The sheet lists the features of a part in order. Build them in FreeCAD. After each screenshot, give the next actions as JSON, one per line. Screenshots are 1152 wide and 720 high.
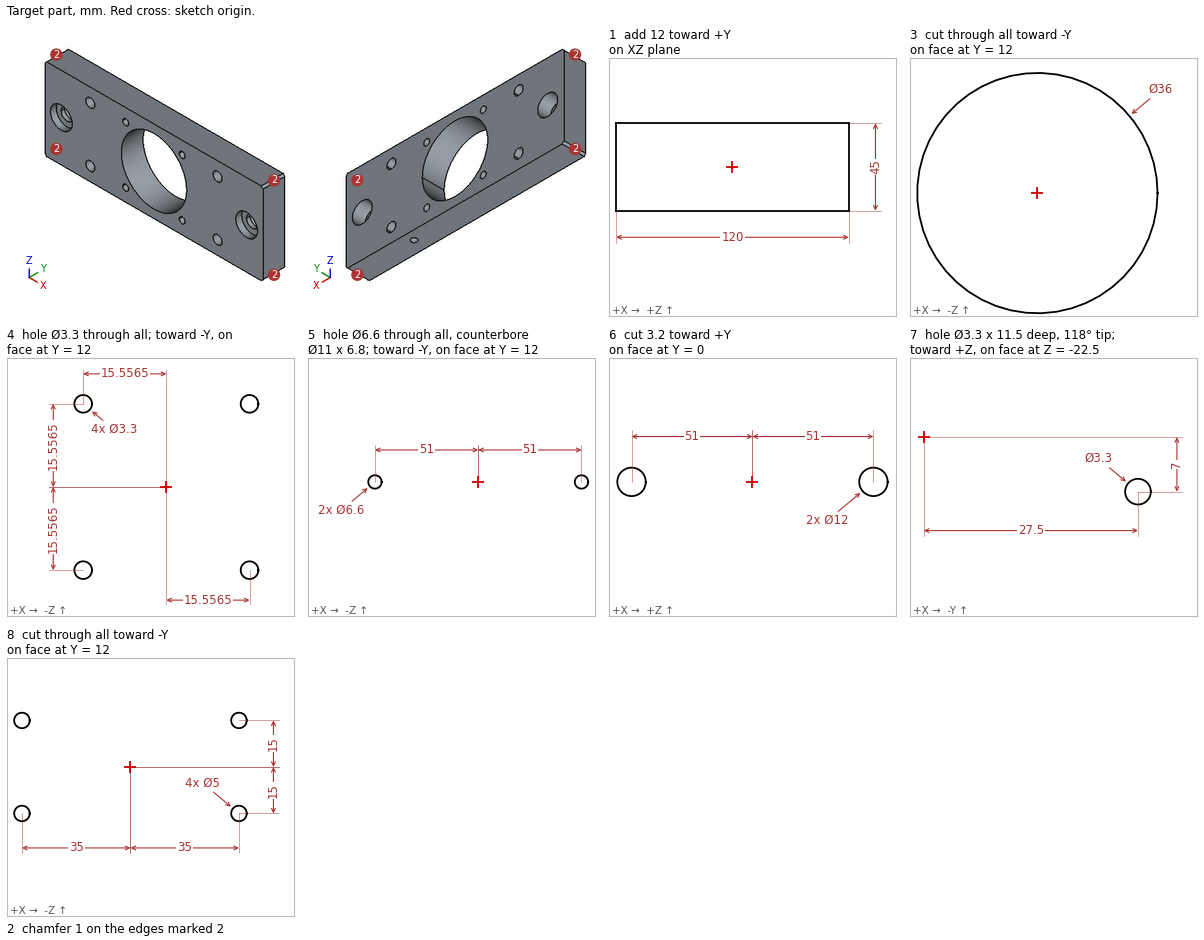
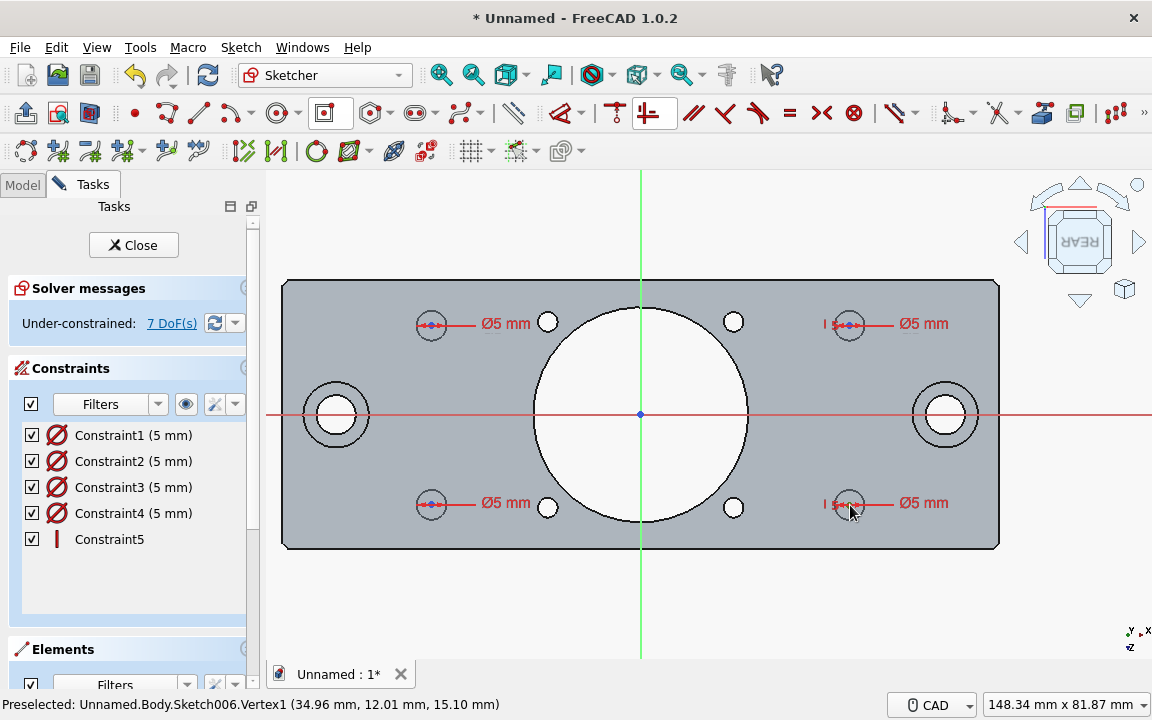
{"action": "left_click", "coordinate": [432, 505]}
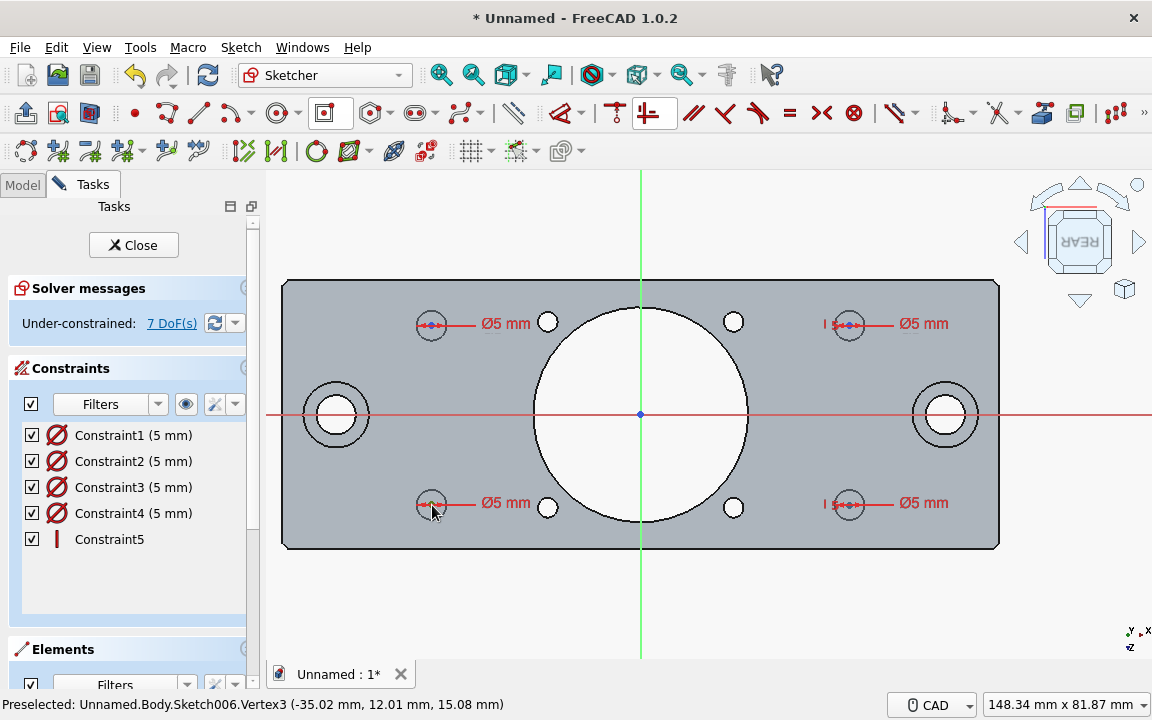
{"action": "key", "text": "h"}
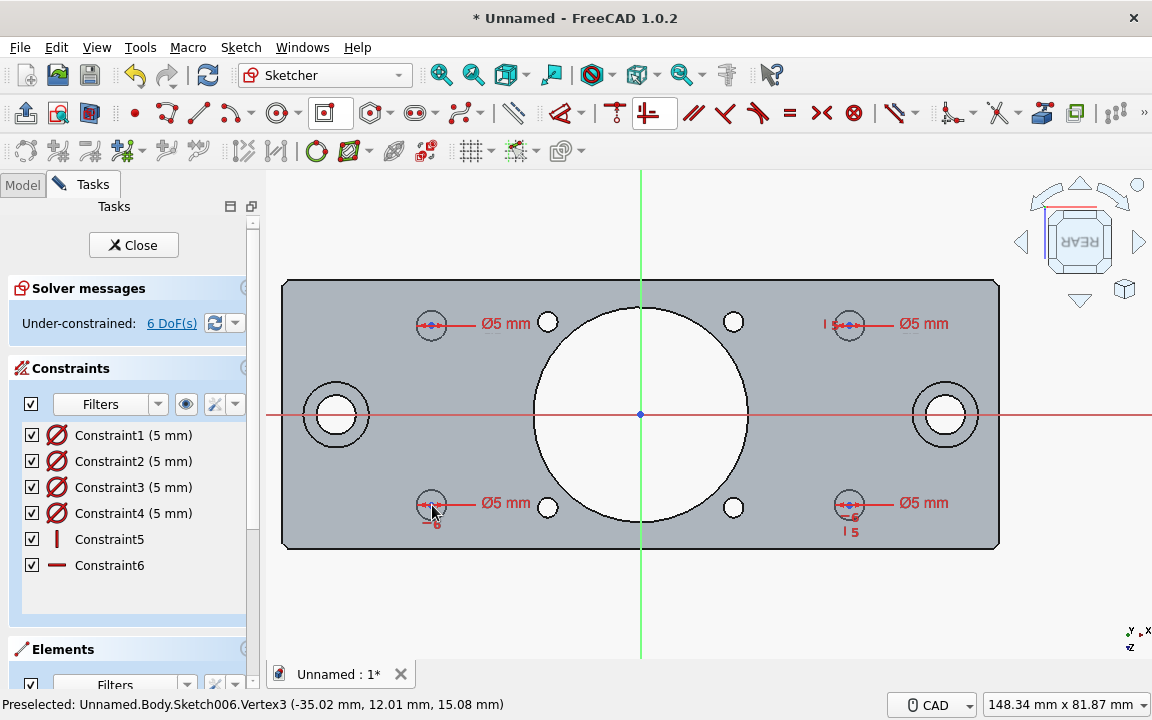
{"action": "left_click", "coordinate": [432, 505]}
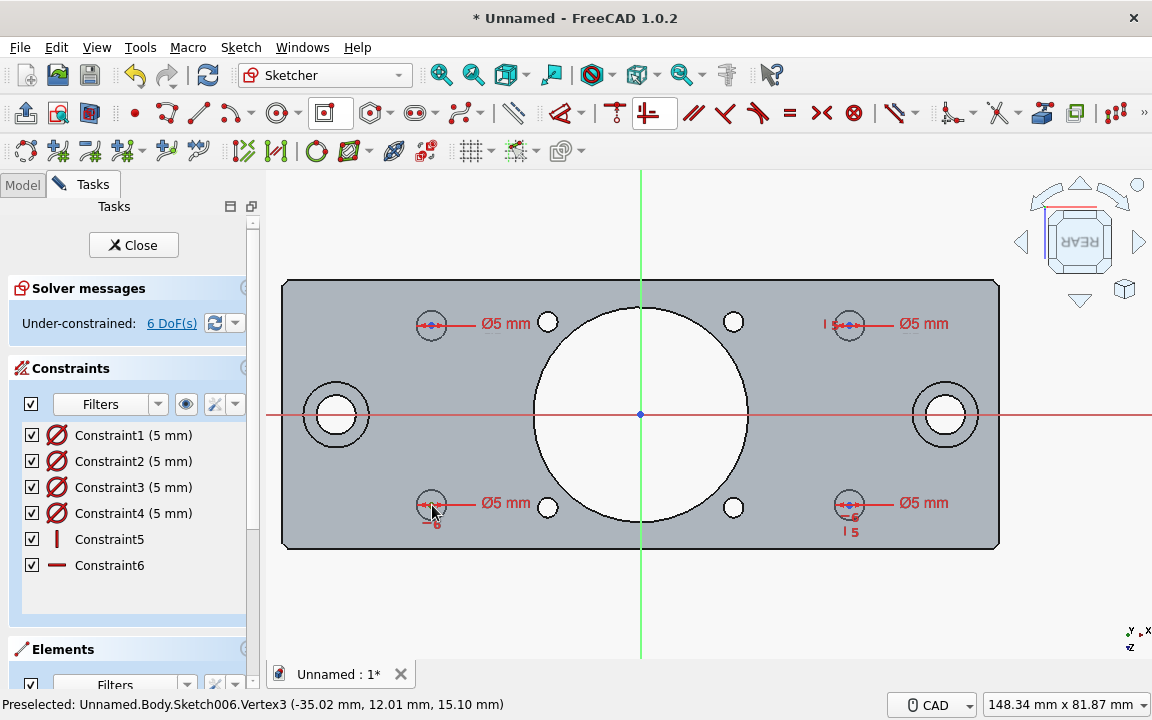
{"action": "left_click", "coordinate": [432, 326]}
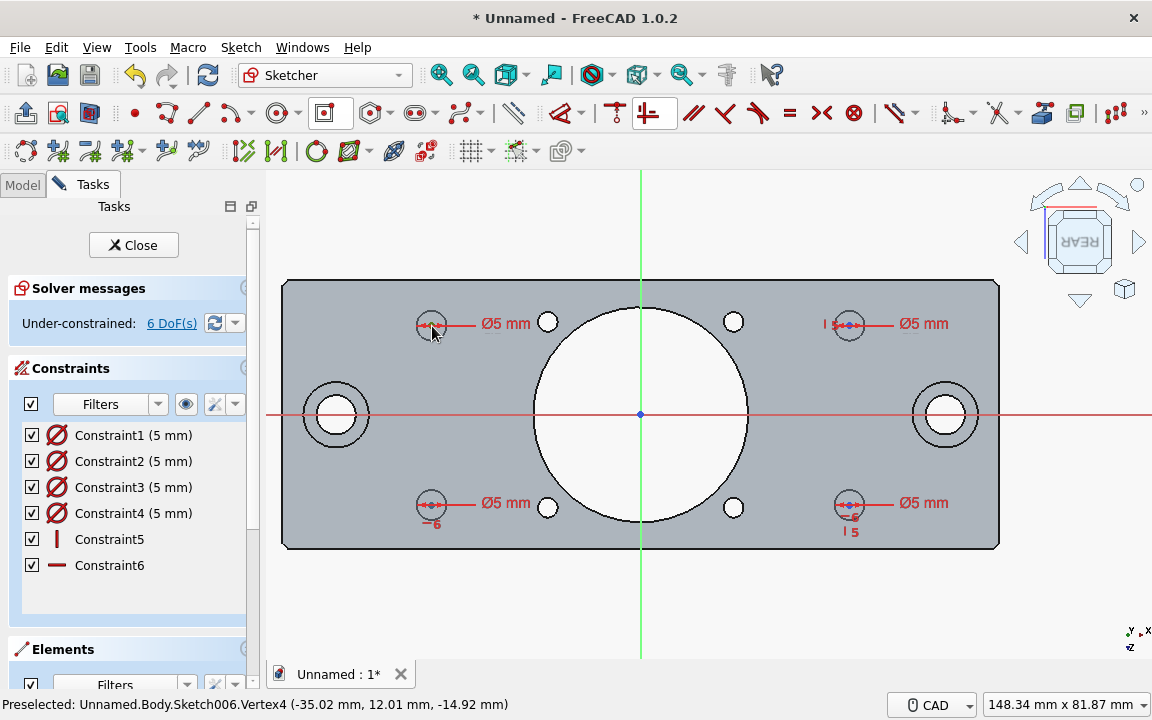
{"action": "key", "text": "v"}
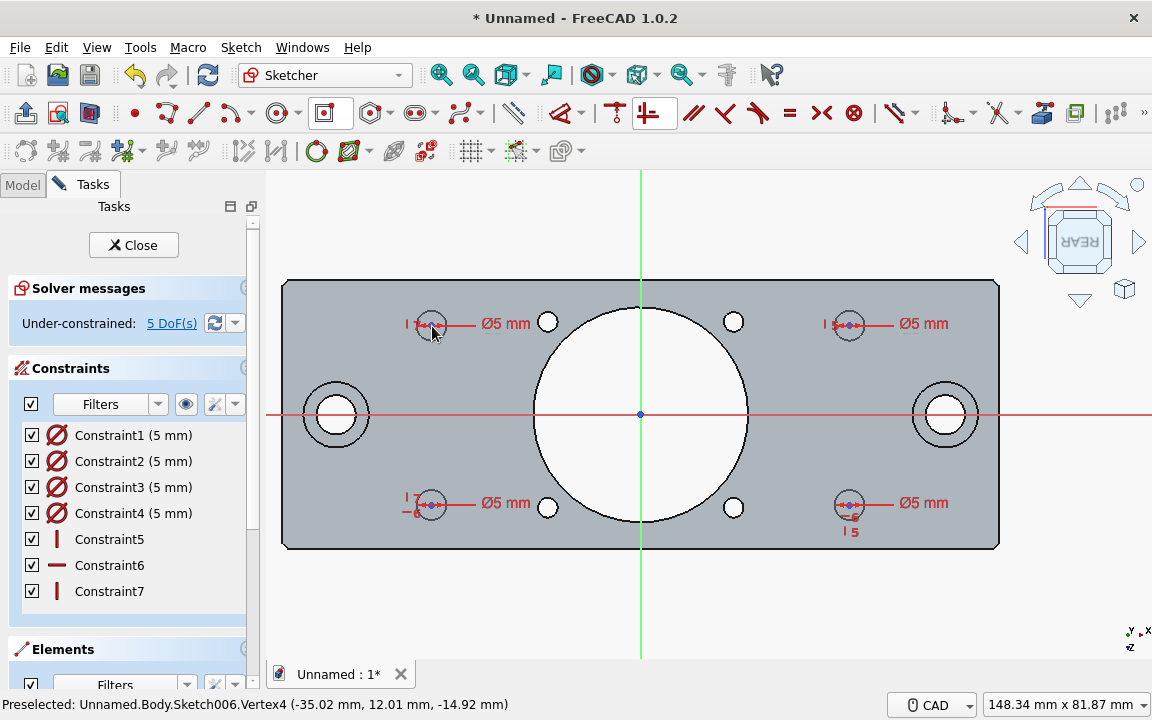
{"action": "left_click", "coordinate": [850, 326]}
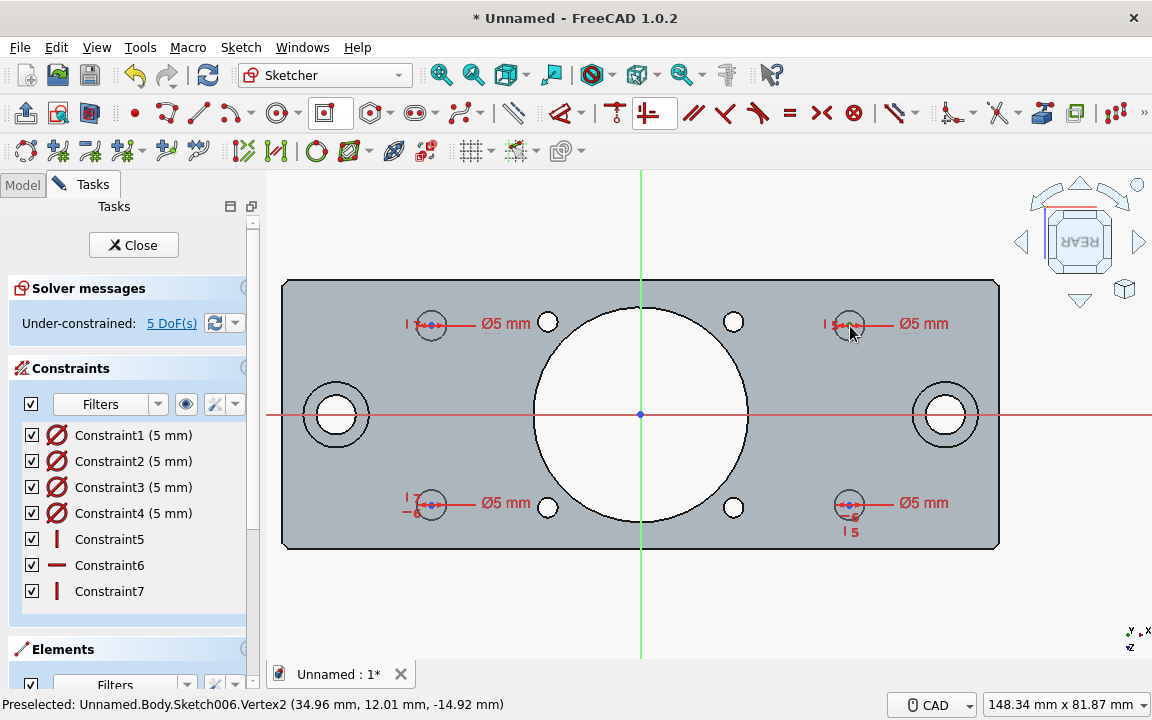
{"action": "left_click", "coordinate": [432, 326]}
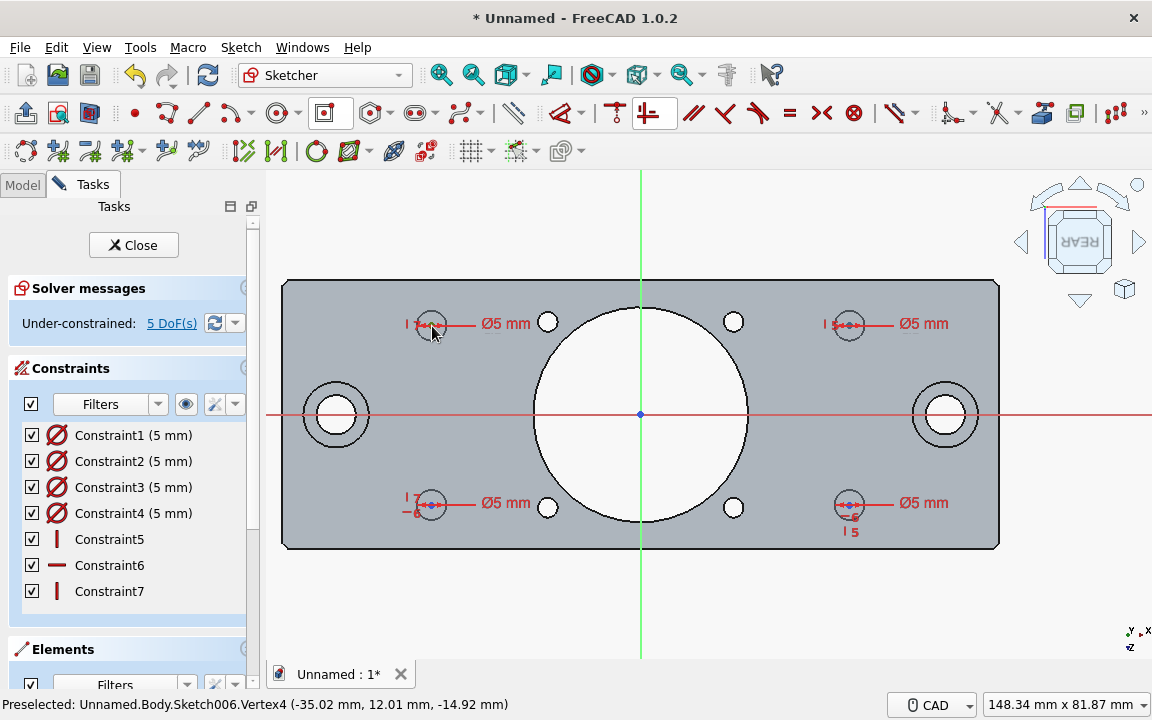
{"action": "left_click", "coordinate": [672, 114]}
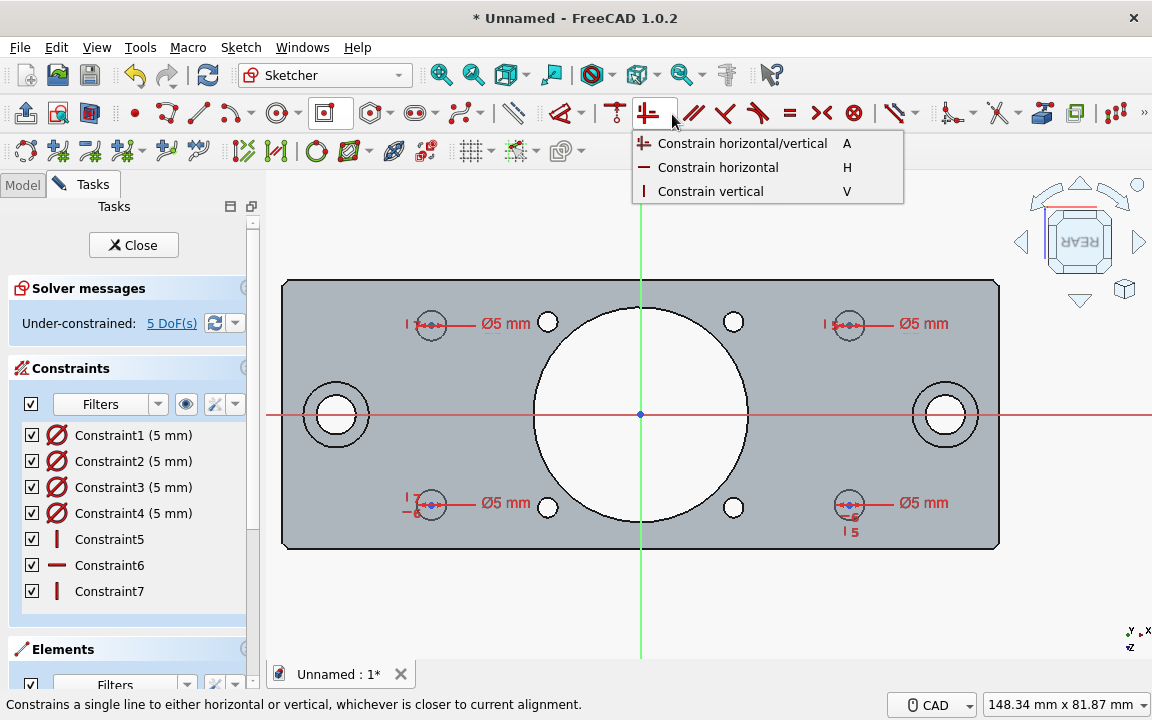
{"action": "left_click", "coordinate": [768, 167]}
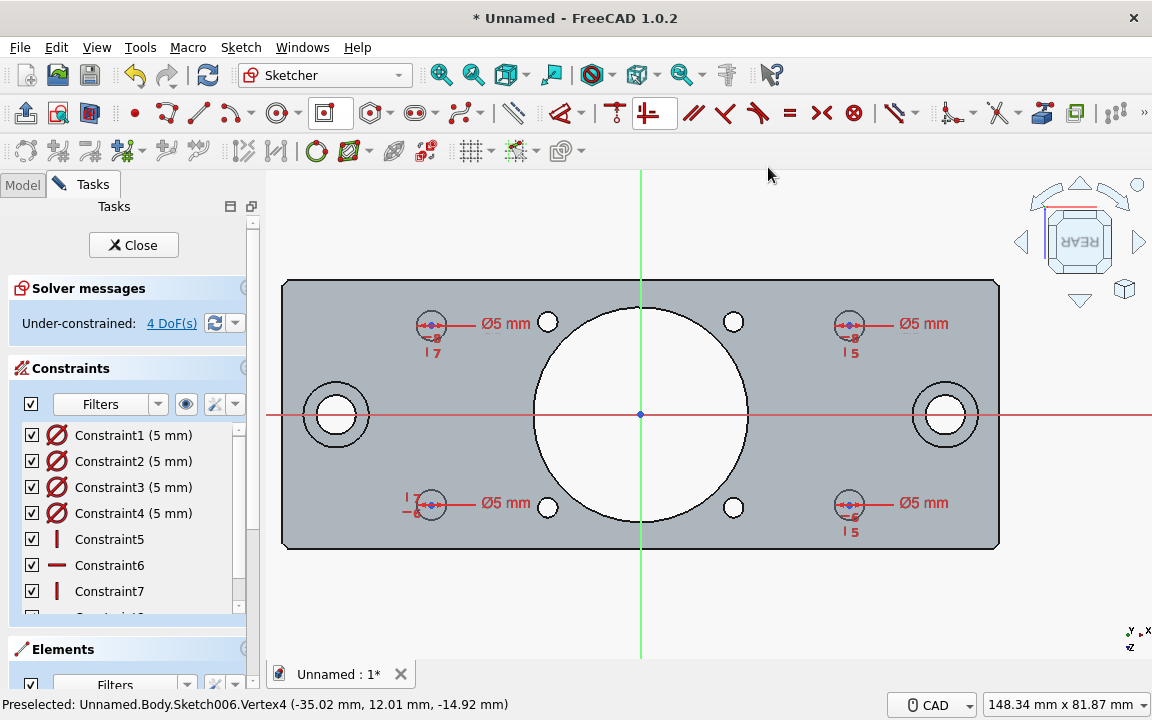
{"action": "left_click", "coordinate": [560, 114]}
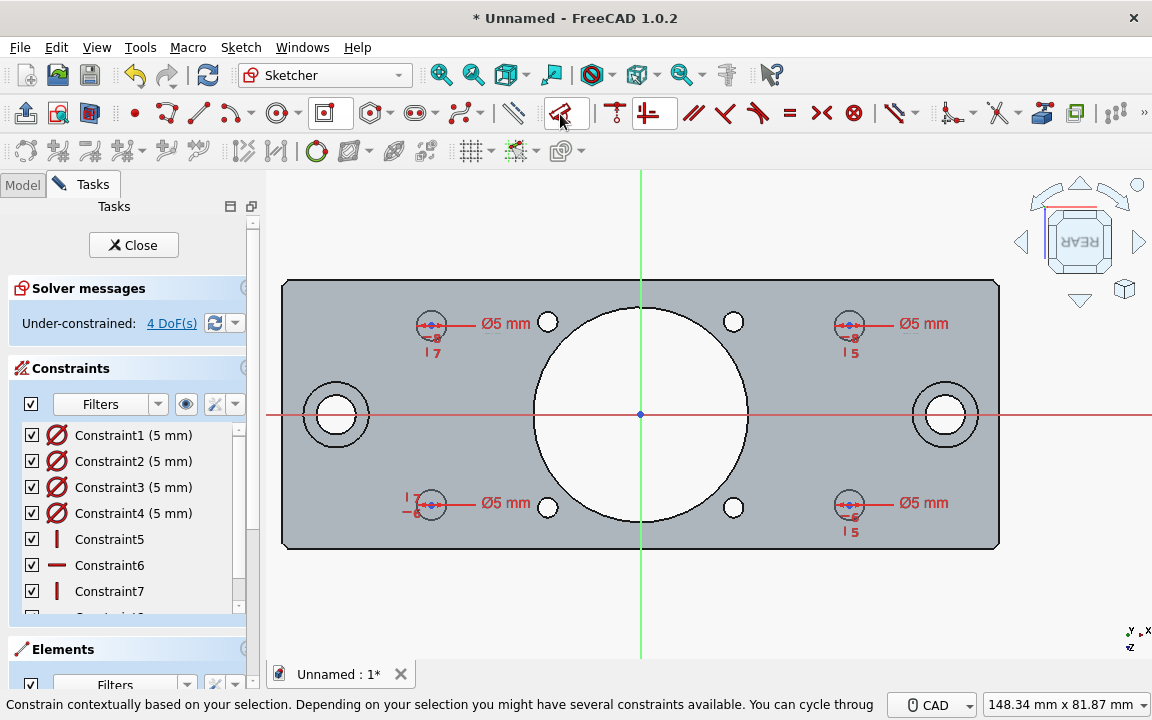
{"action": "left_click", "coordinate": [850, 505]}
{"action": "left_click", "coordinate": [745, 539]}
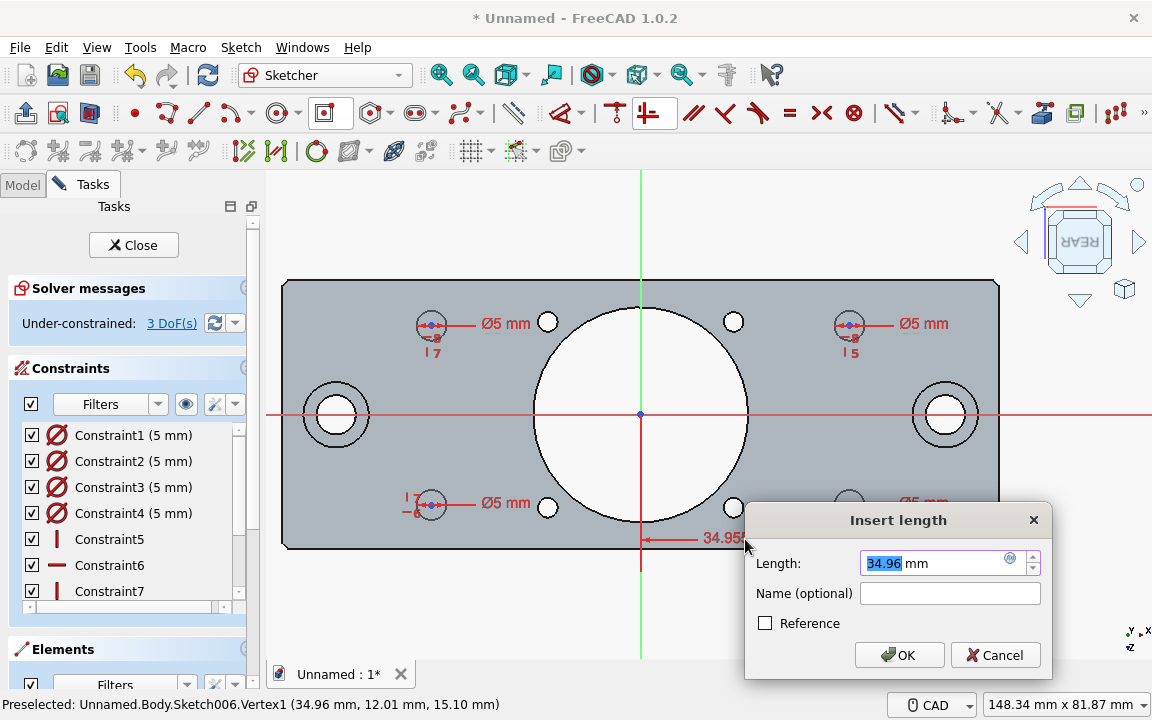
{"action": "type", "text": "35"}
{"action": "key", "text": "Return"}